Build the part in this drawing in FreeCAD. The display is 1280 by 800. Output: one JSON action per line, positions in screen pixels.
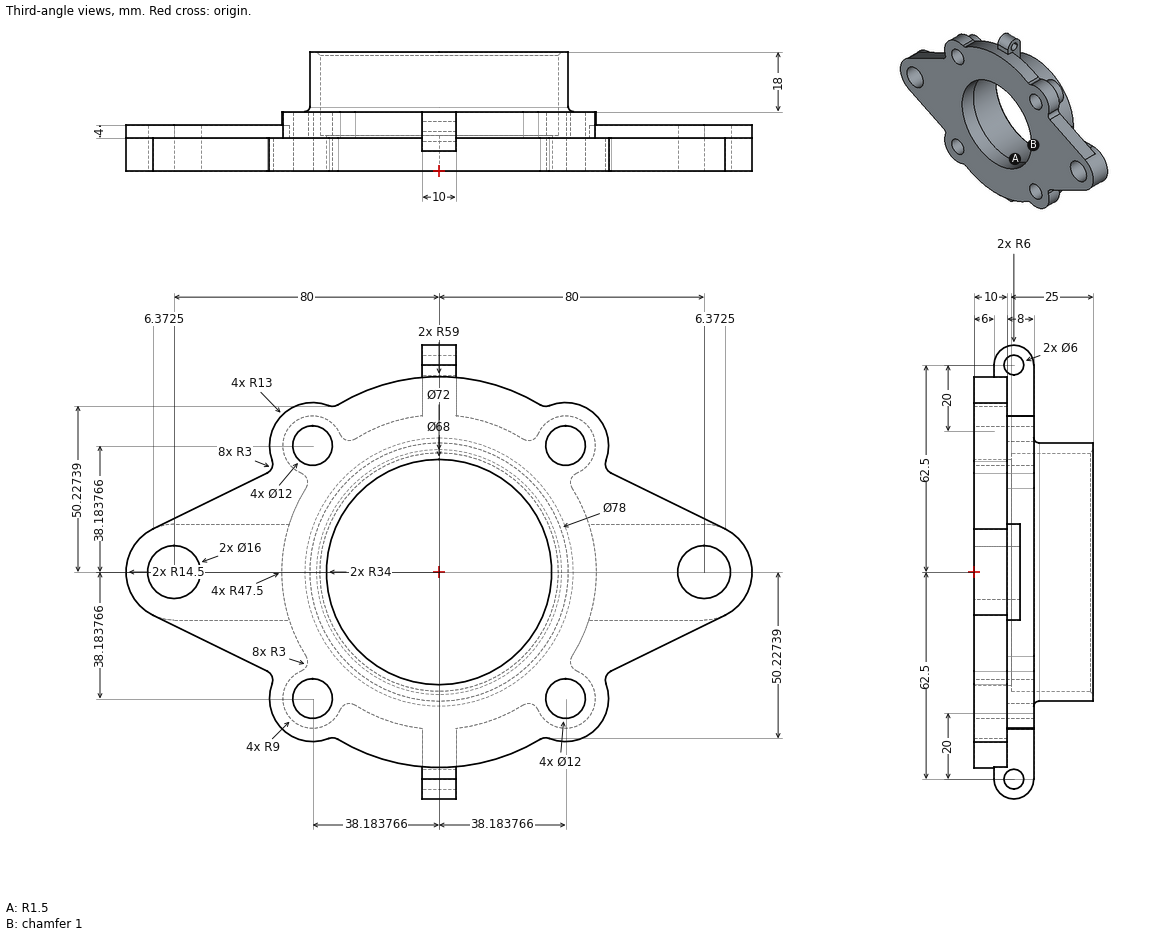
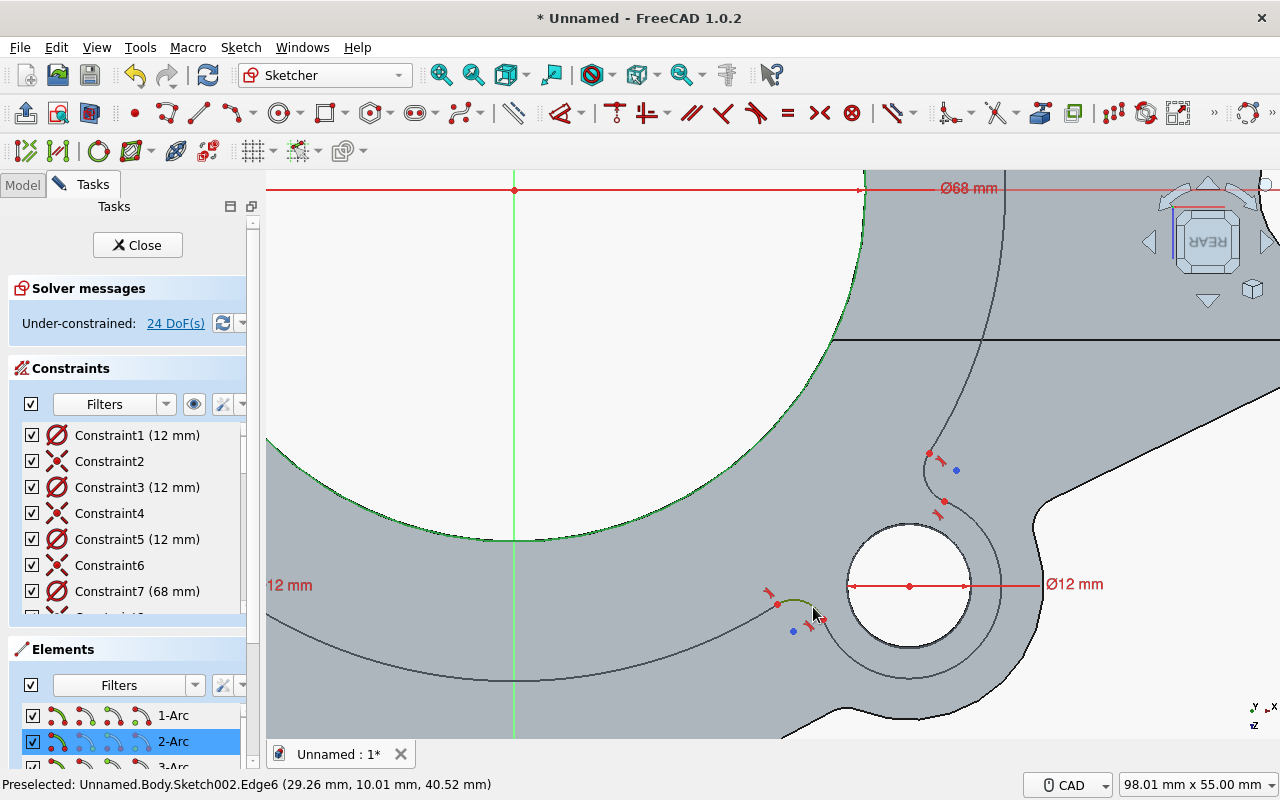
{"action": "left_click", "coordinate": [924, 469]}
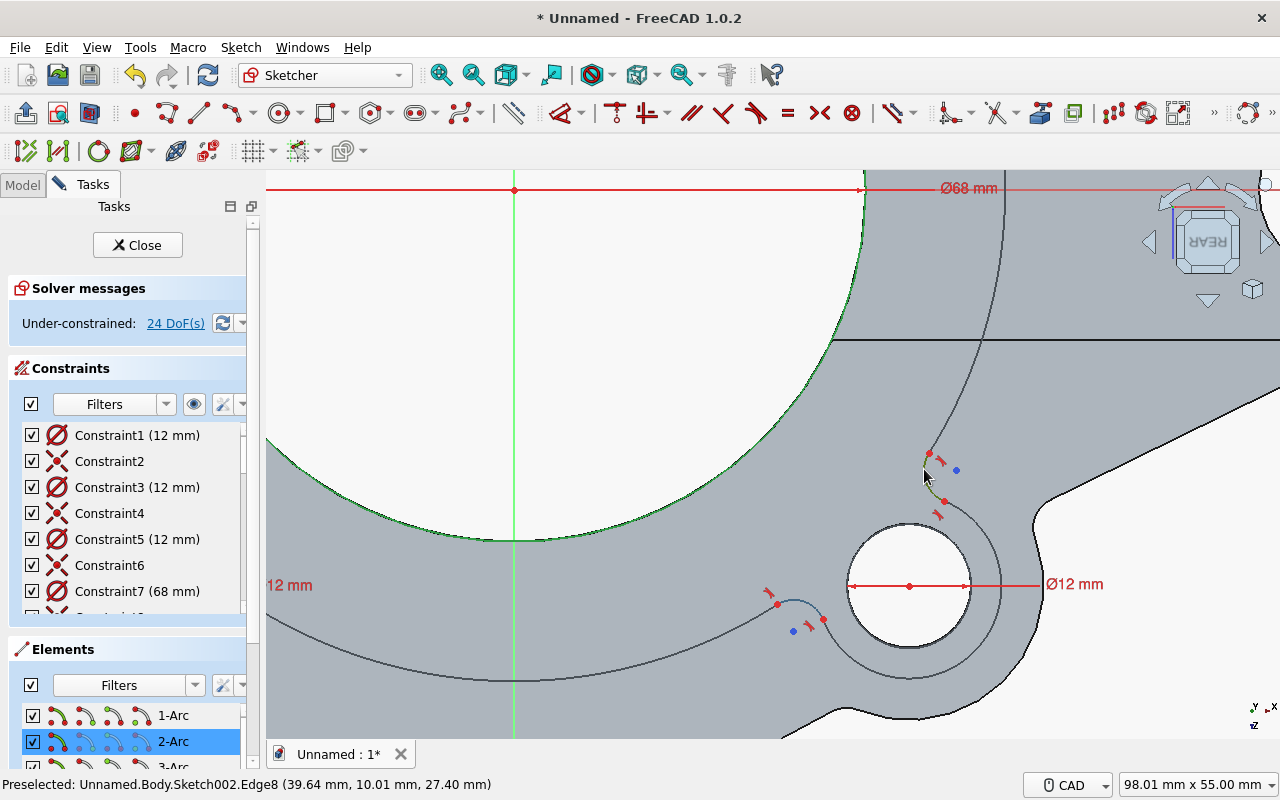
{"action": "scroll", "coordinate": [815, 608], "scroll_direction": "down", "scroll_amount": 5}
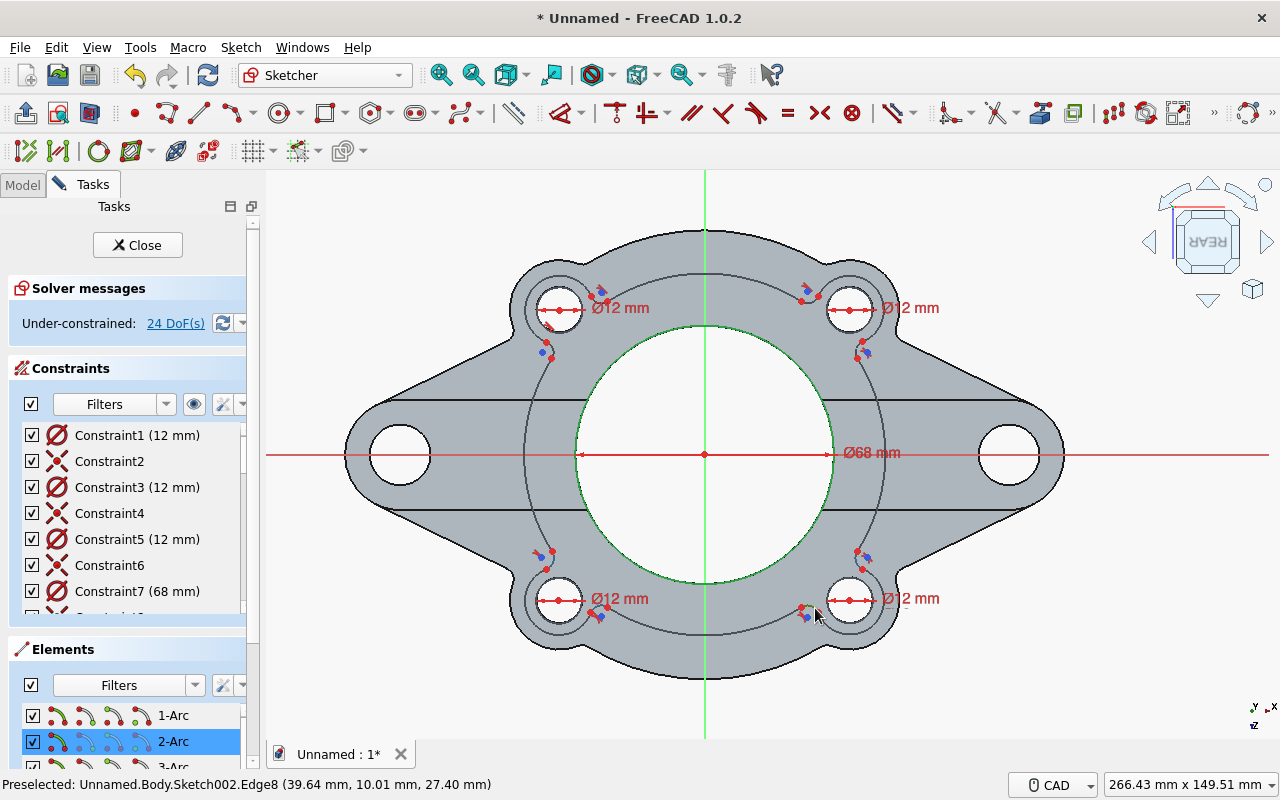
{"action": "scroll", "coordinate": [858, 345], "scroll_direction": "up", "scroll_amount": 5}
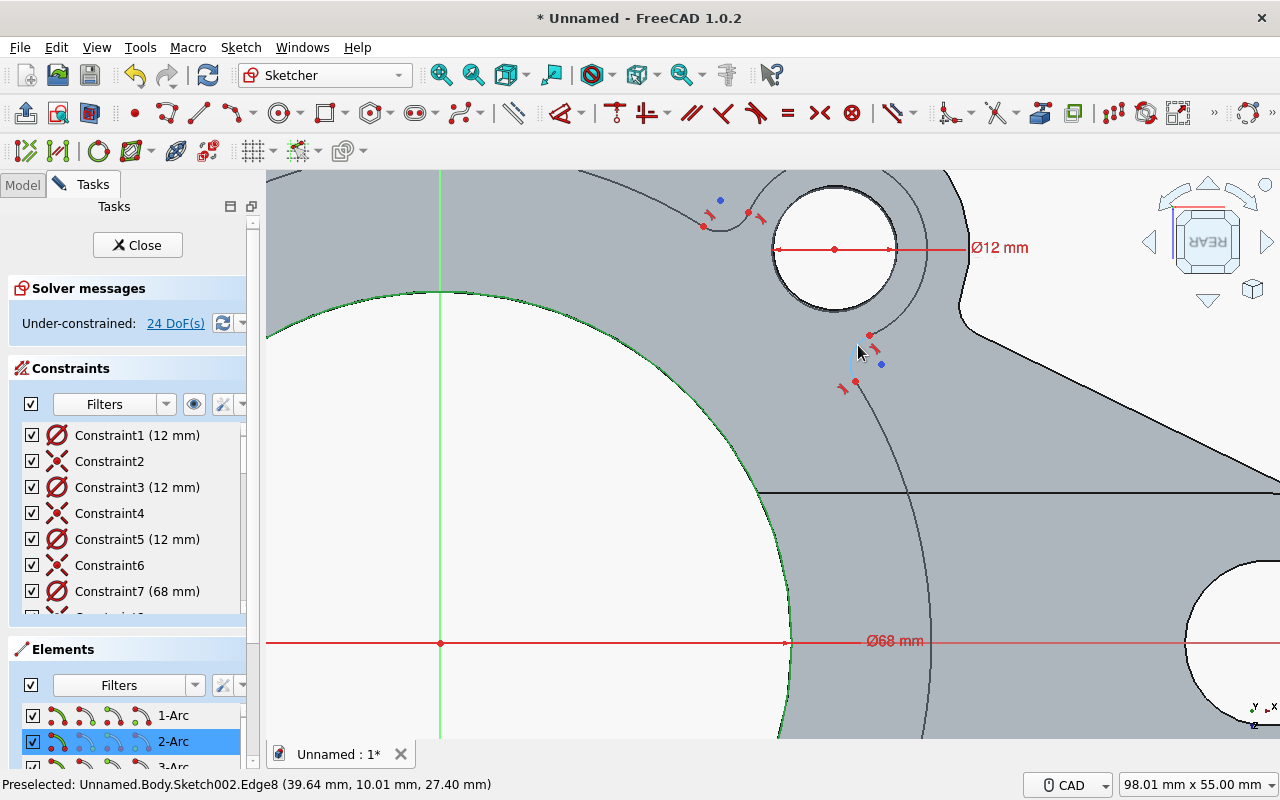
{"action": "left_click", "coordinate": [857, 345]}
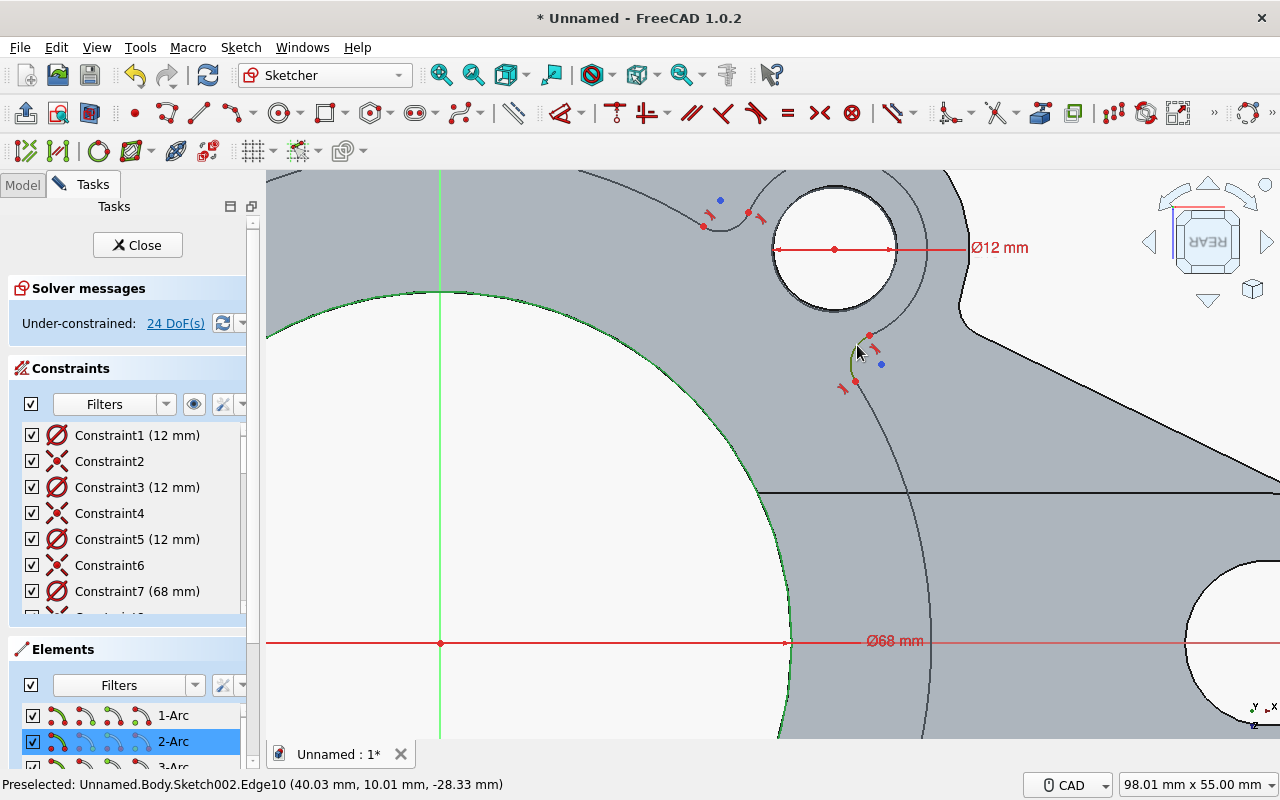
{"action": "left_click", "coordinate": [719, 231]}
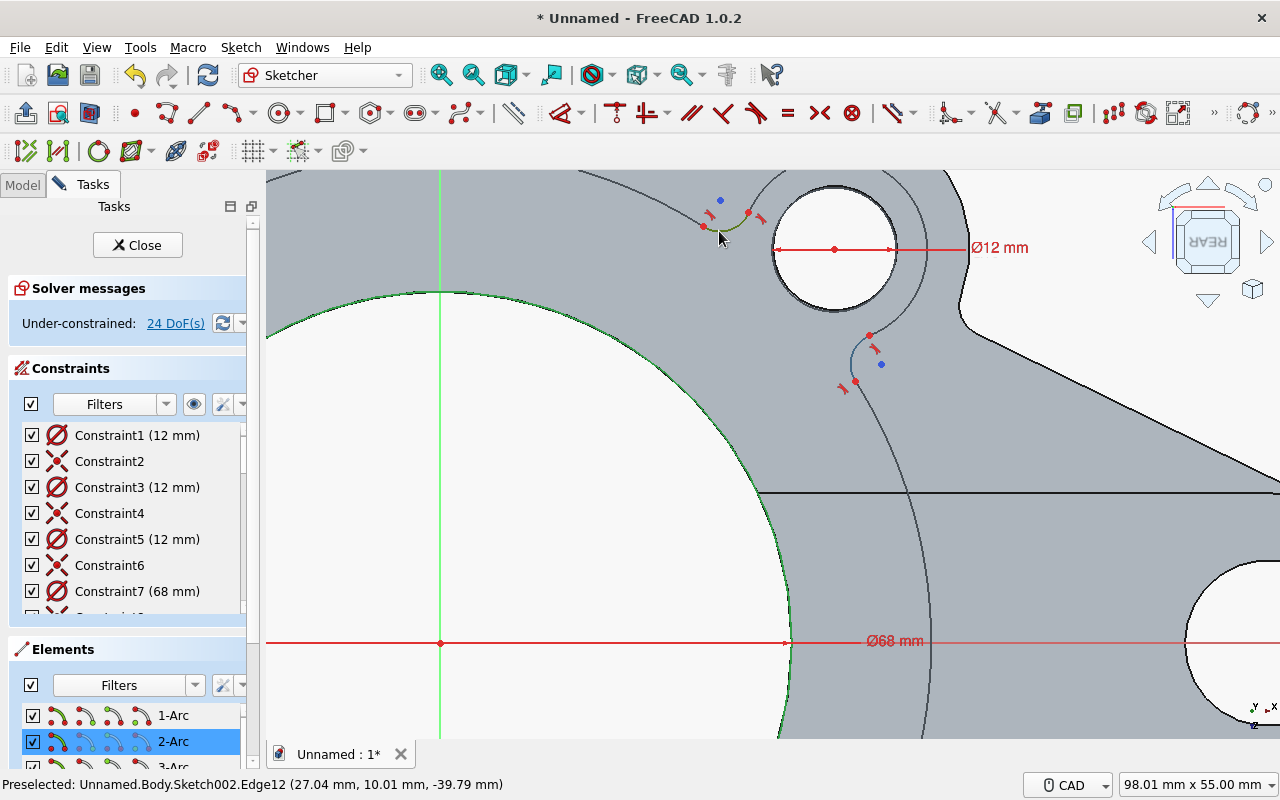
{"action": "scroll", "coordinate": [858, 345], "scroll_direction": "down", "scroll_amount": 5}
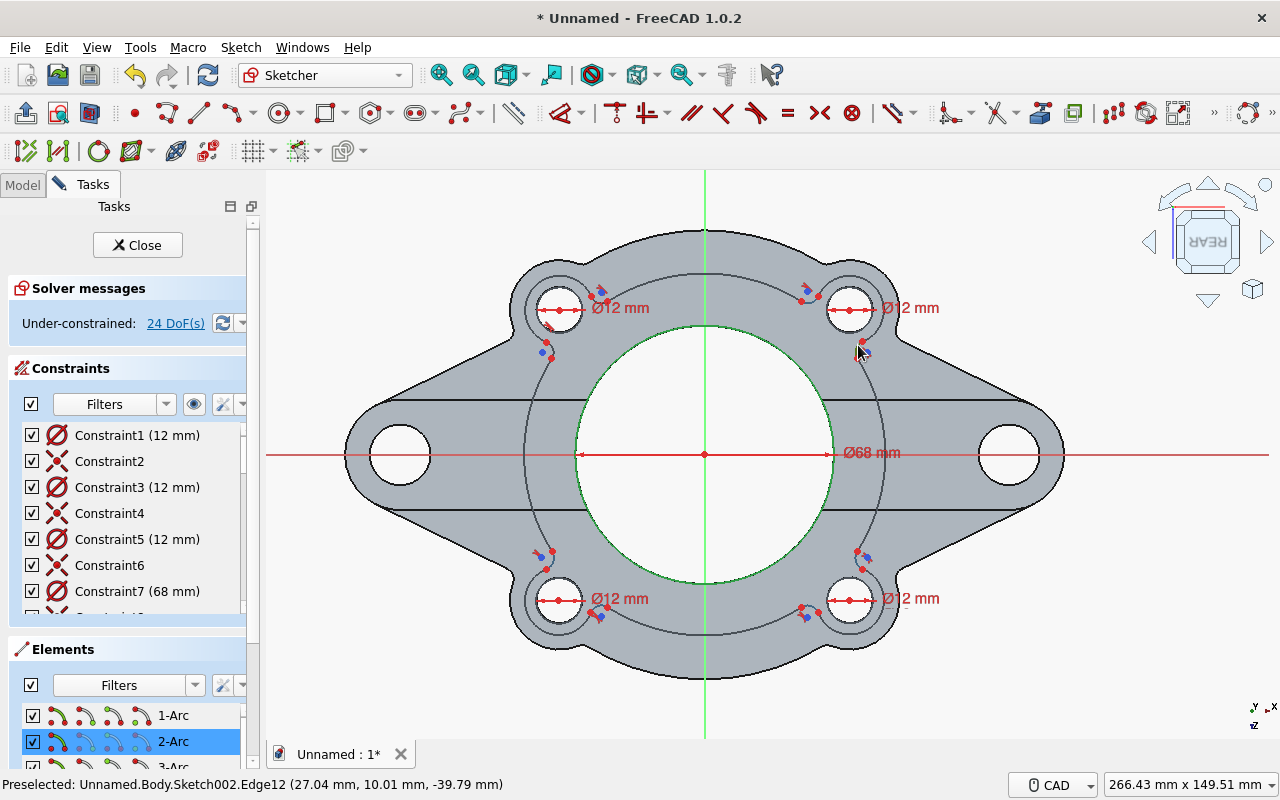
{"action": "scroll", "coordinate": [595, 301], "scroll_direction": "up", "scroll_amount": 5}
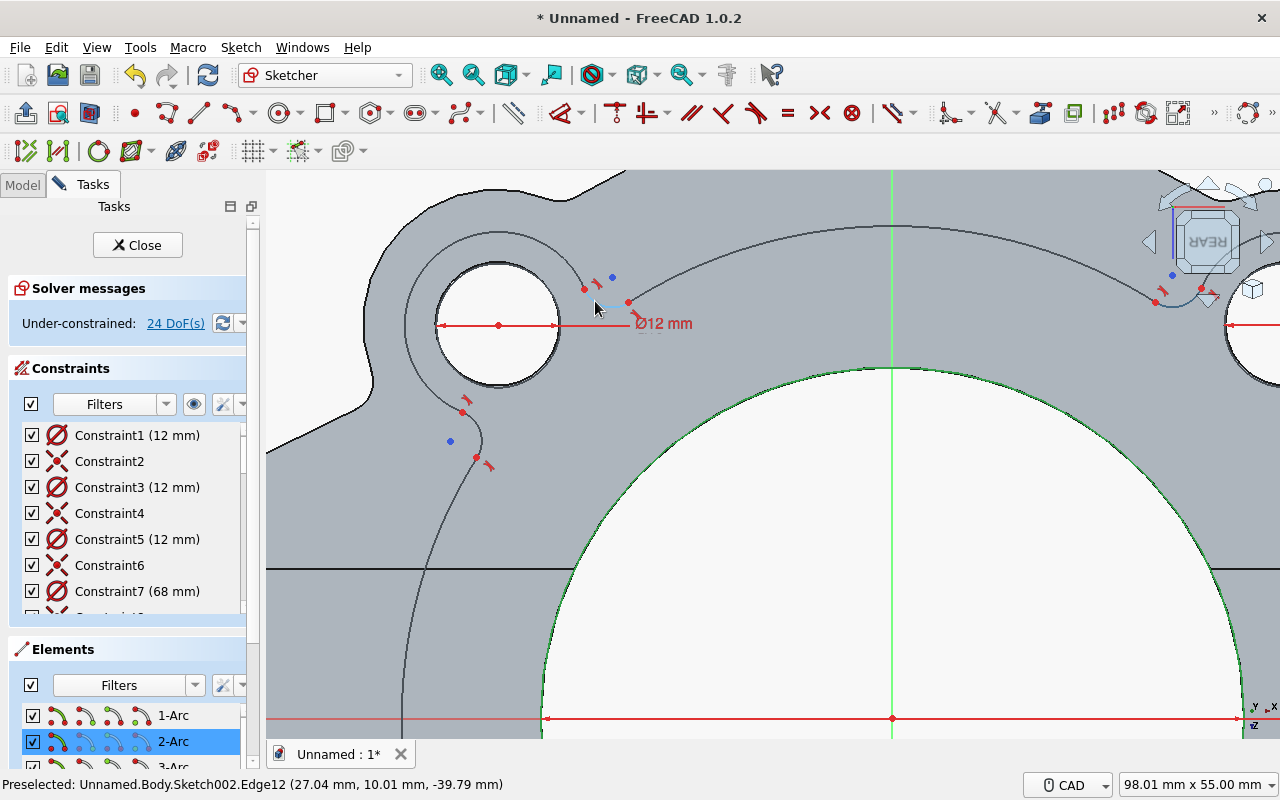
{"action": "left_click", "coordinate": [594, 301]}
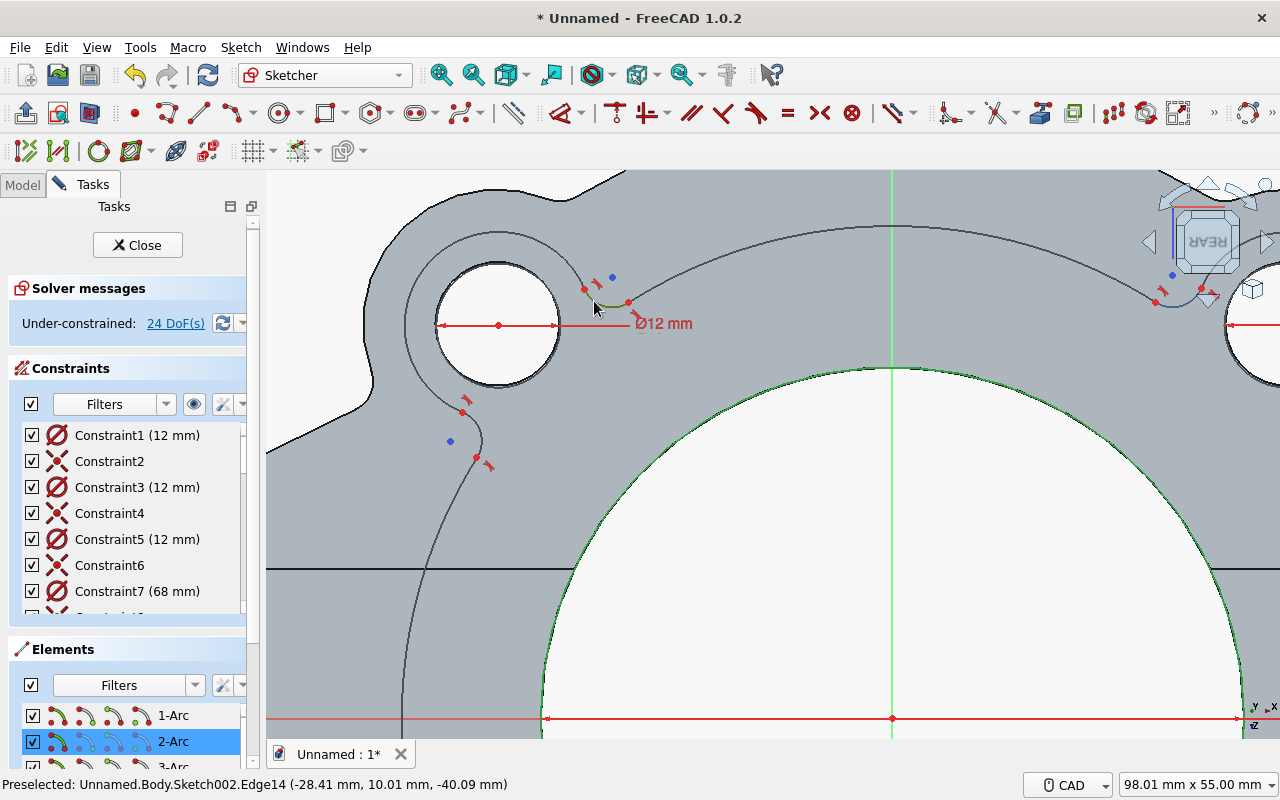
{"action": "left_click", "coordinate": [482, 442]}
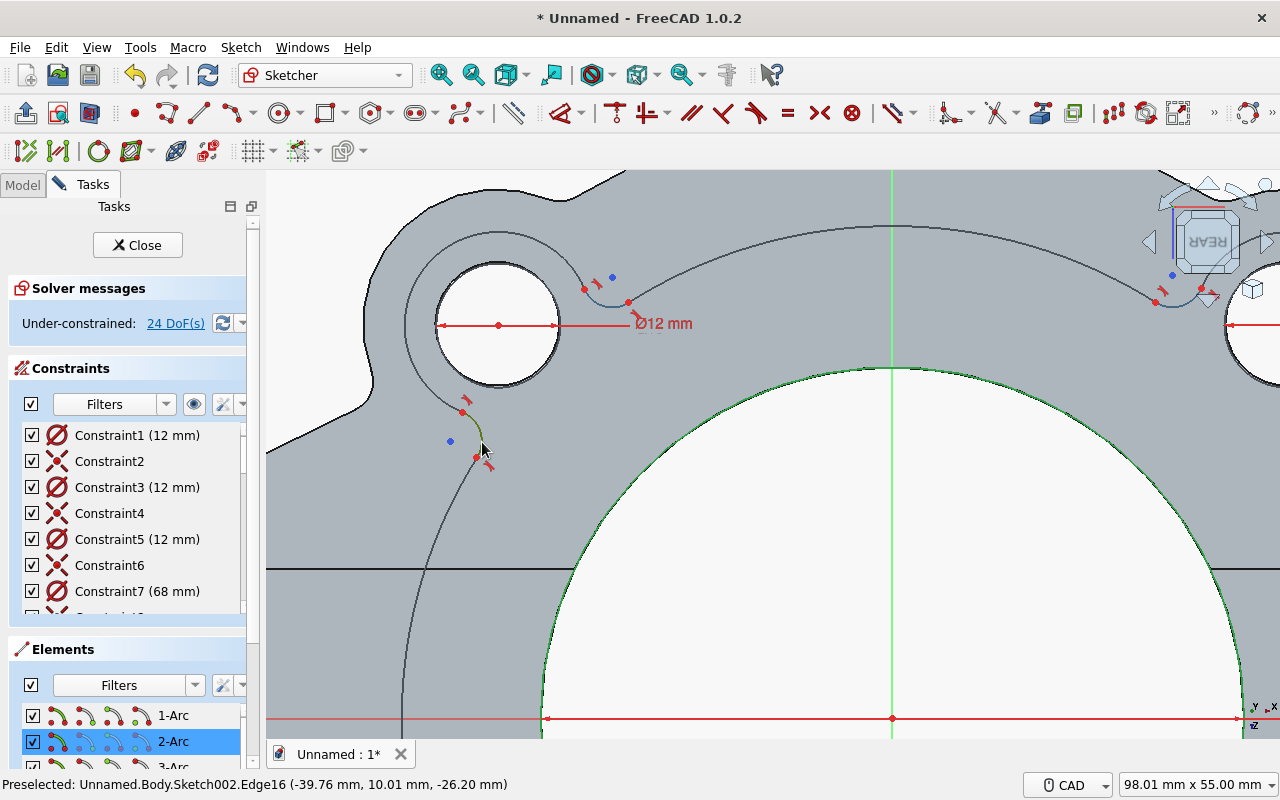
{"action": "left_click", "coordinate": [788, 114]}